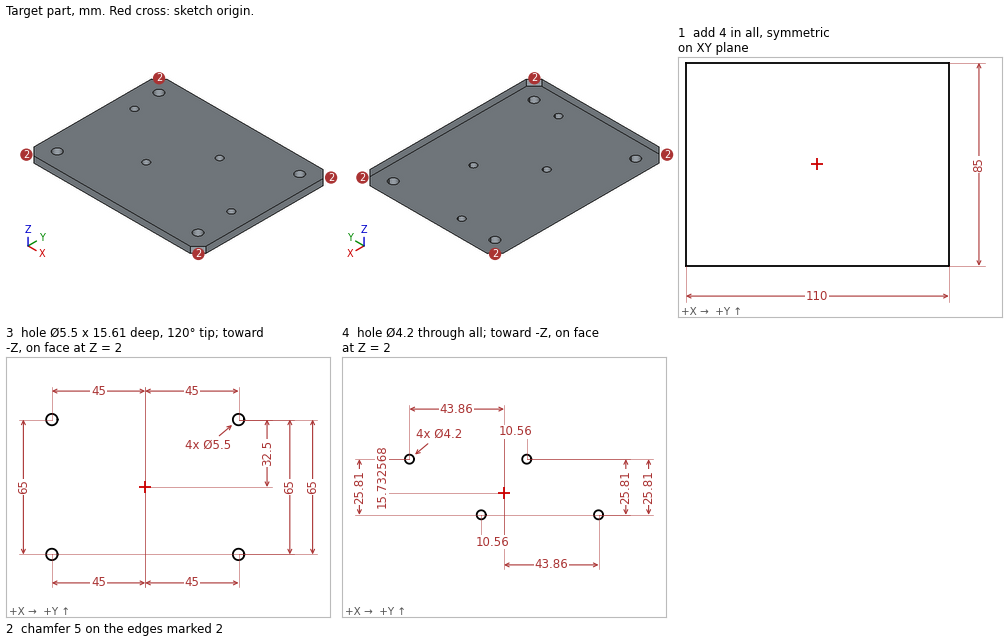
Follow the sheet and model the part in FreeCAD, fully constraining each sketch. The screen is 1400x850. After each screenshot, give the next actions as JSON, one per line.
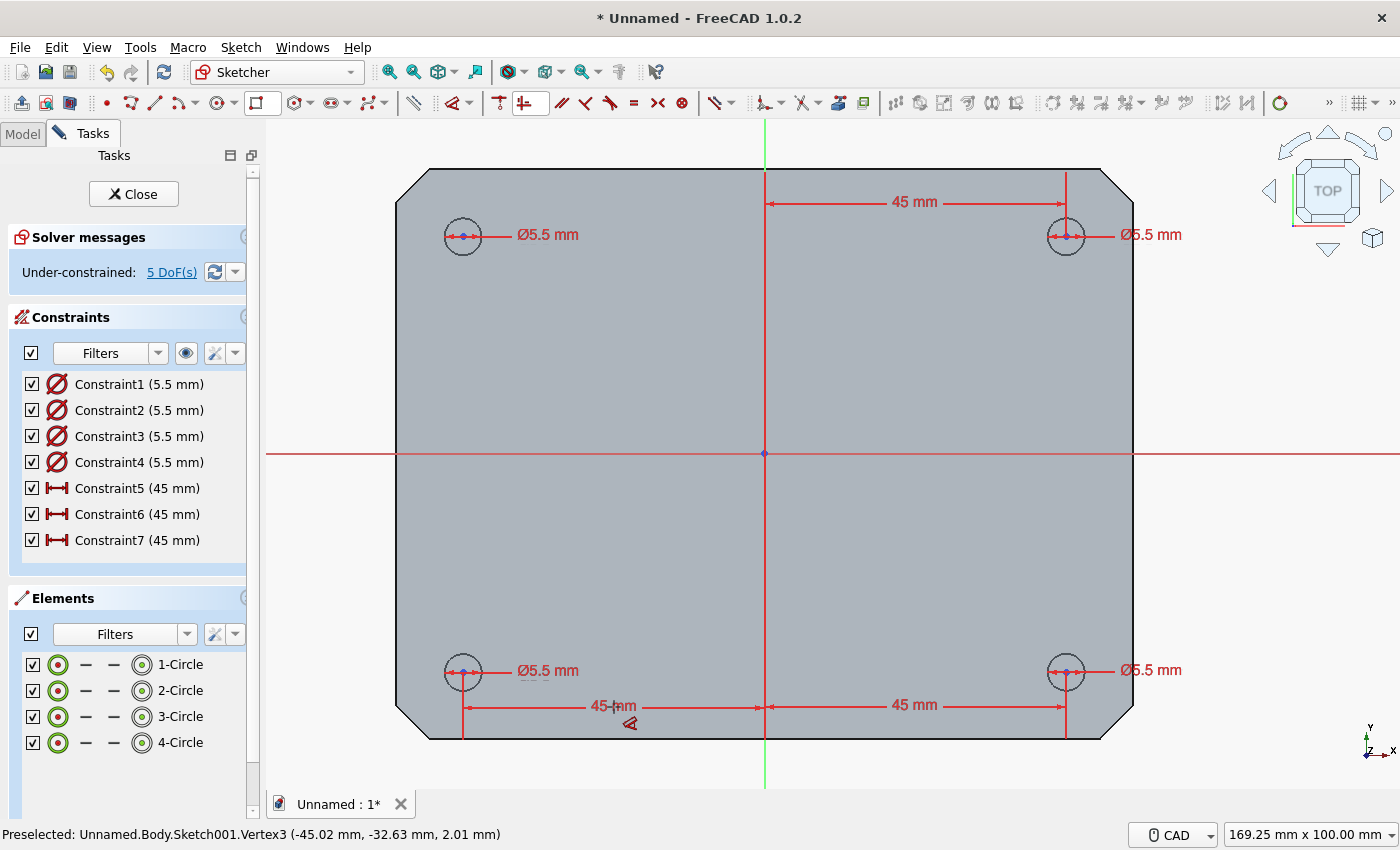
{"action": "left_click", "coordinate": [463, 237]}
{"action": "left_click", "coordinate": [614, 203]}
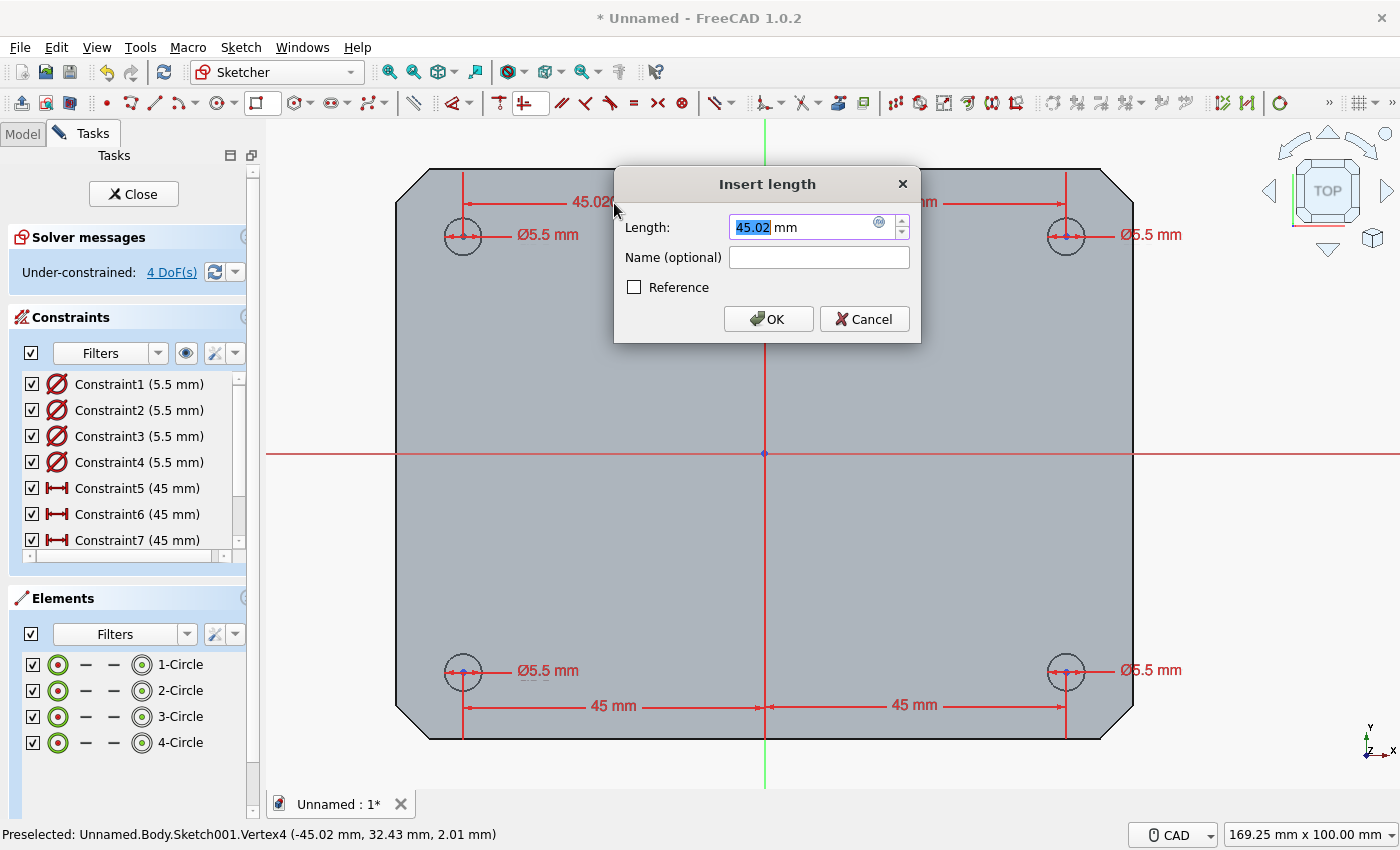
{"action": "type", "text": "45"}
{"action": "key", "text": "Return"}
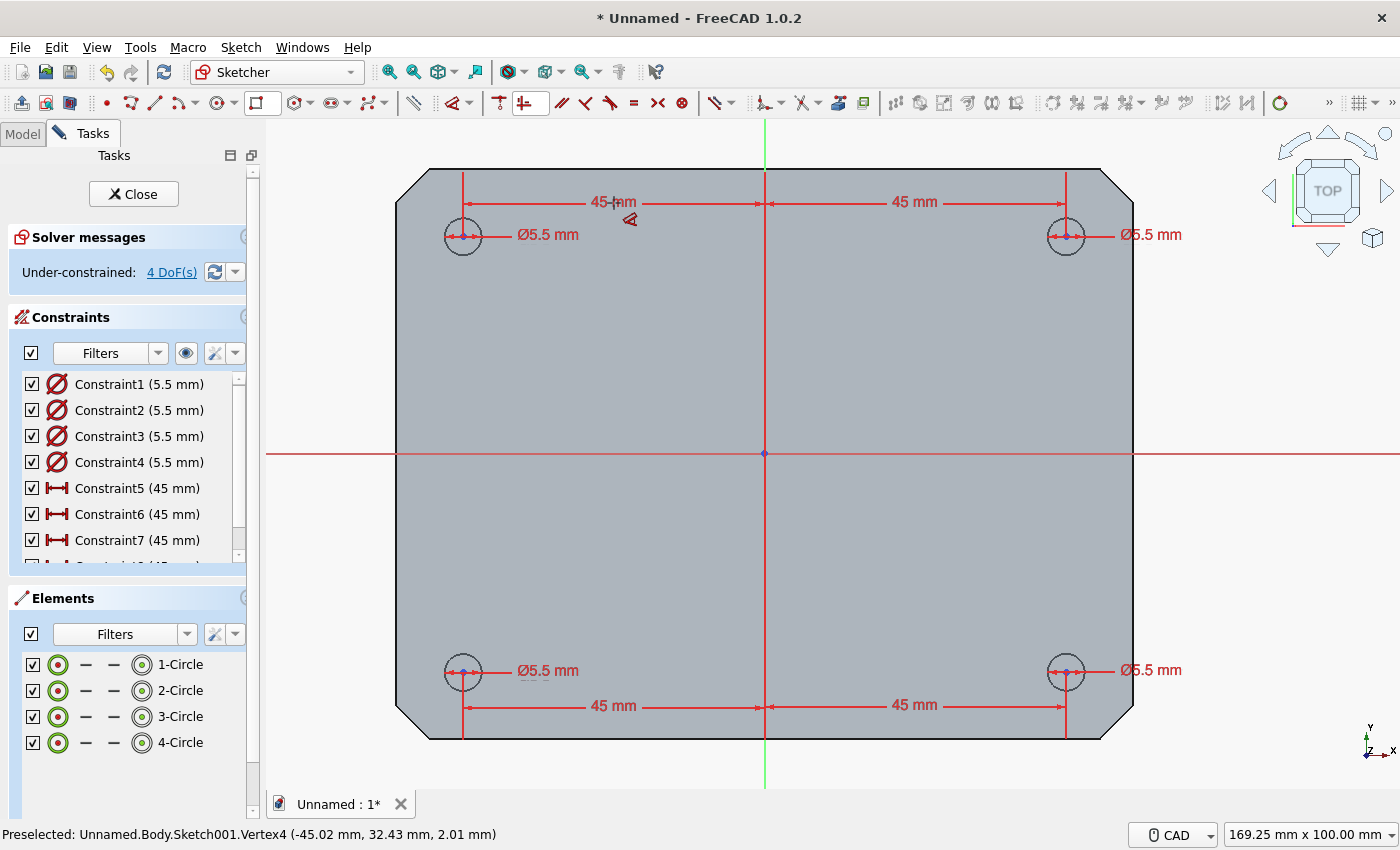
{"action": "left_click", "coordinate": [1066, 237]}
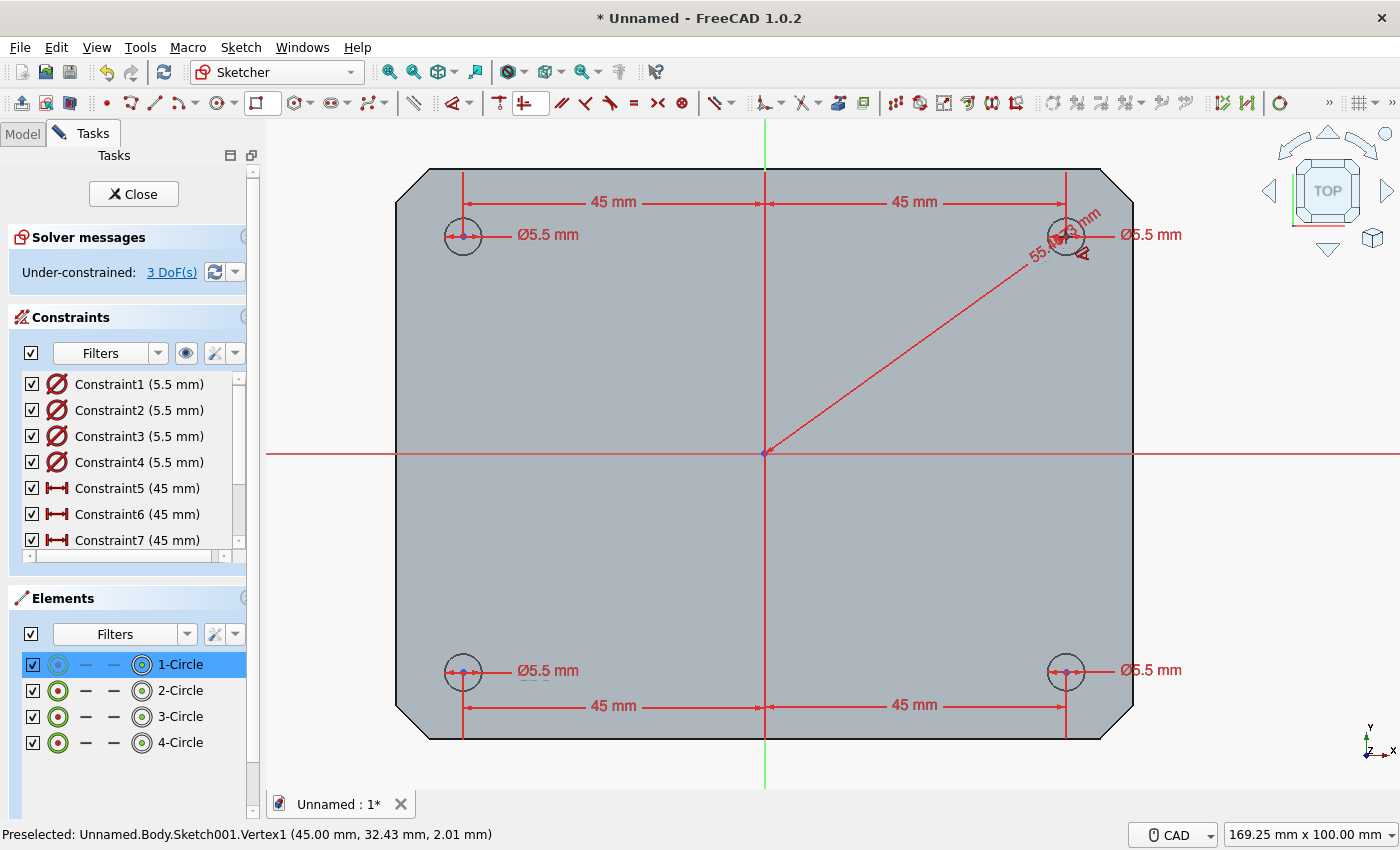
{"action": "left_click", "coordinate": [1066, 672]}
{"action": "left_click", "coordinate": [1100, 354]}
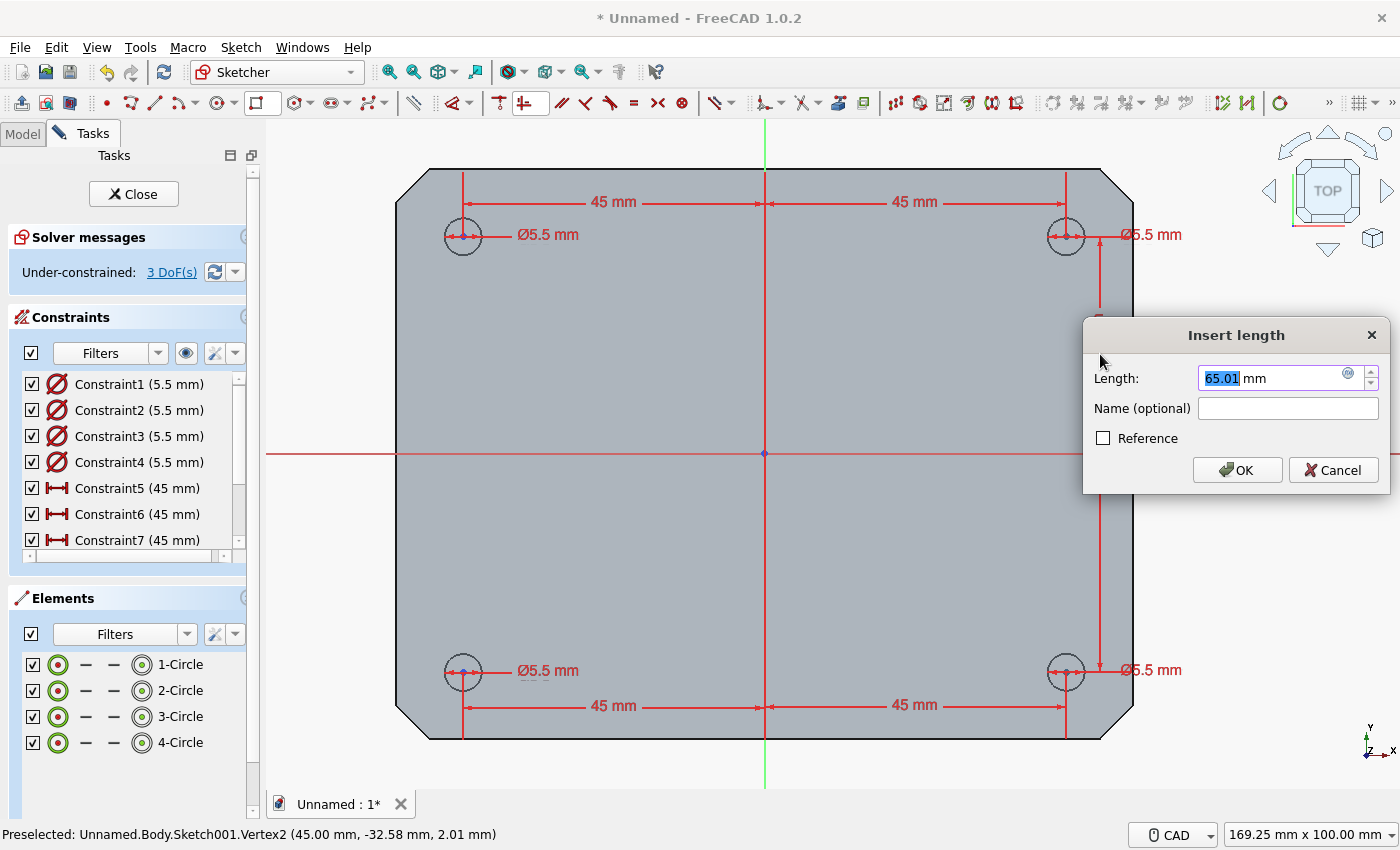
{"action": "type", "text": "65"}
{"action": "key", "text": "Return"}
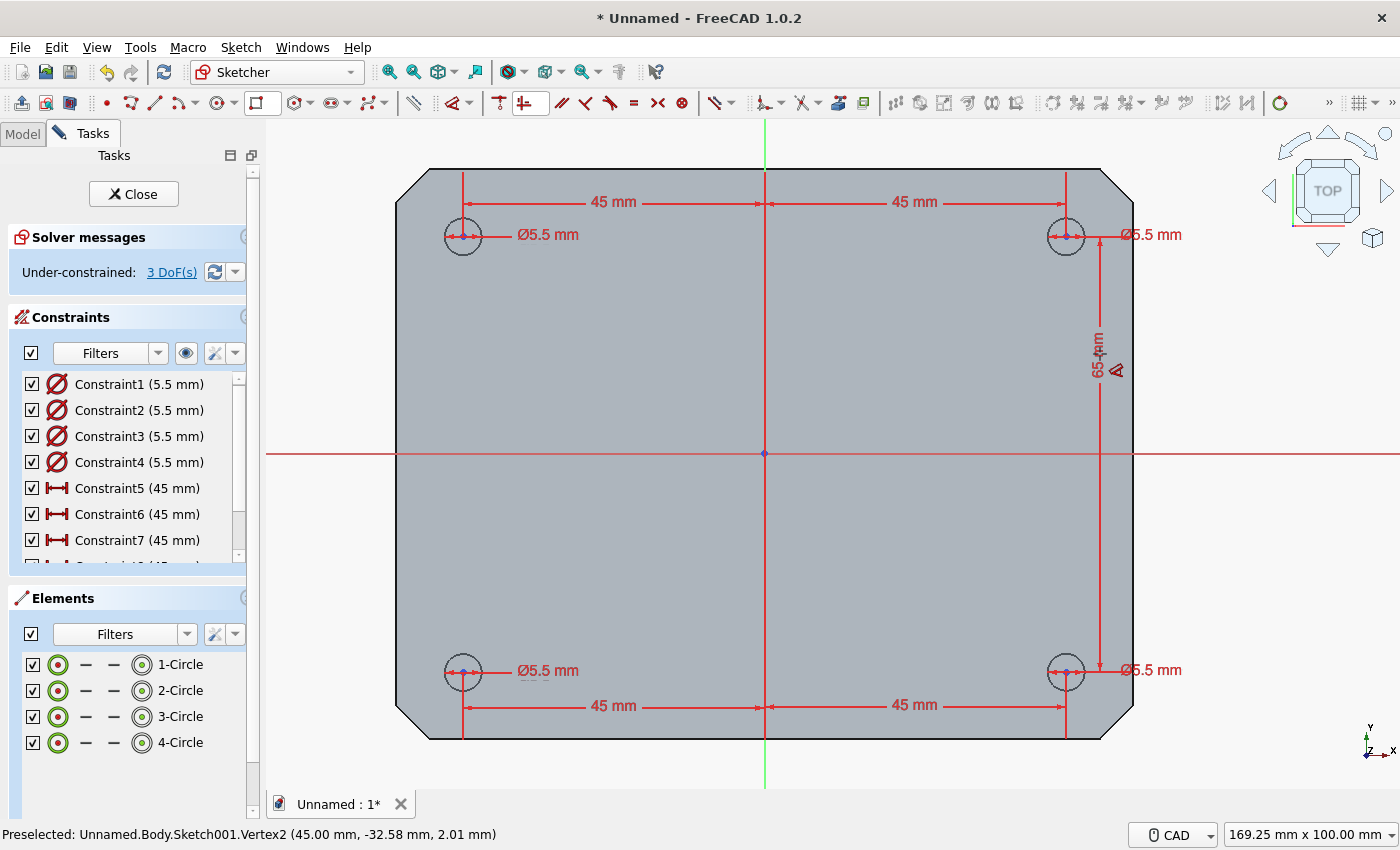
{"action": "left_click", "coordinate": [1066, 237]}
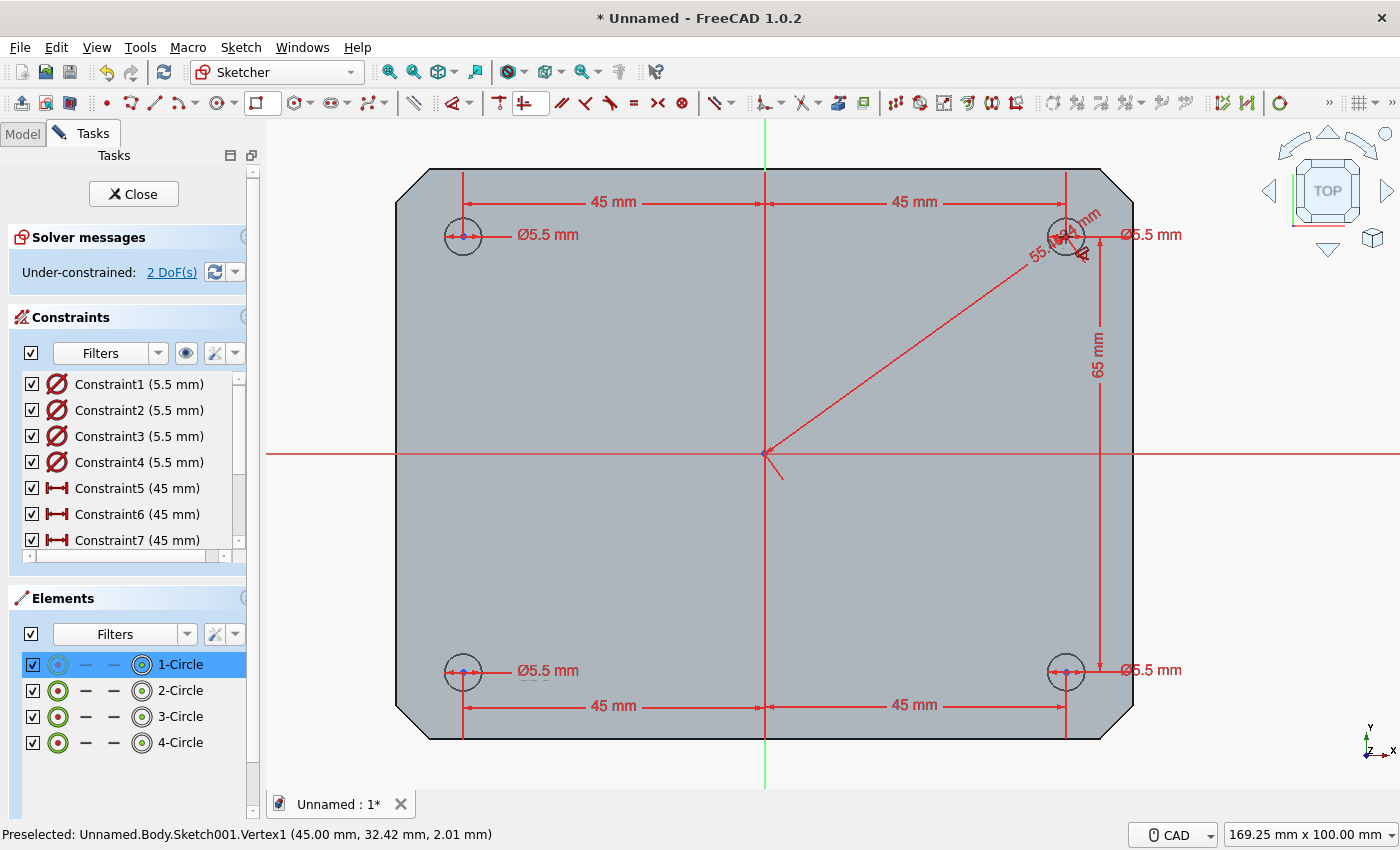
{"action": "left_click", "coordinate": [463, 673]}
{"action": "left_click", "coordinate": [429, 354]}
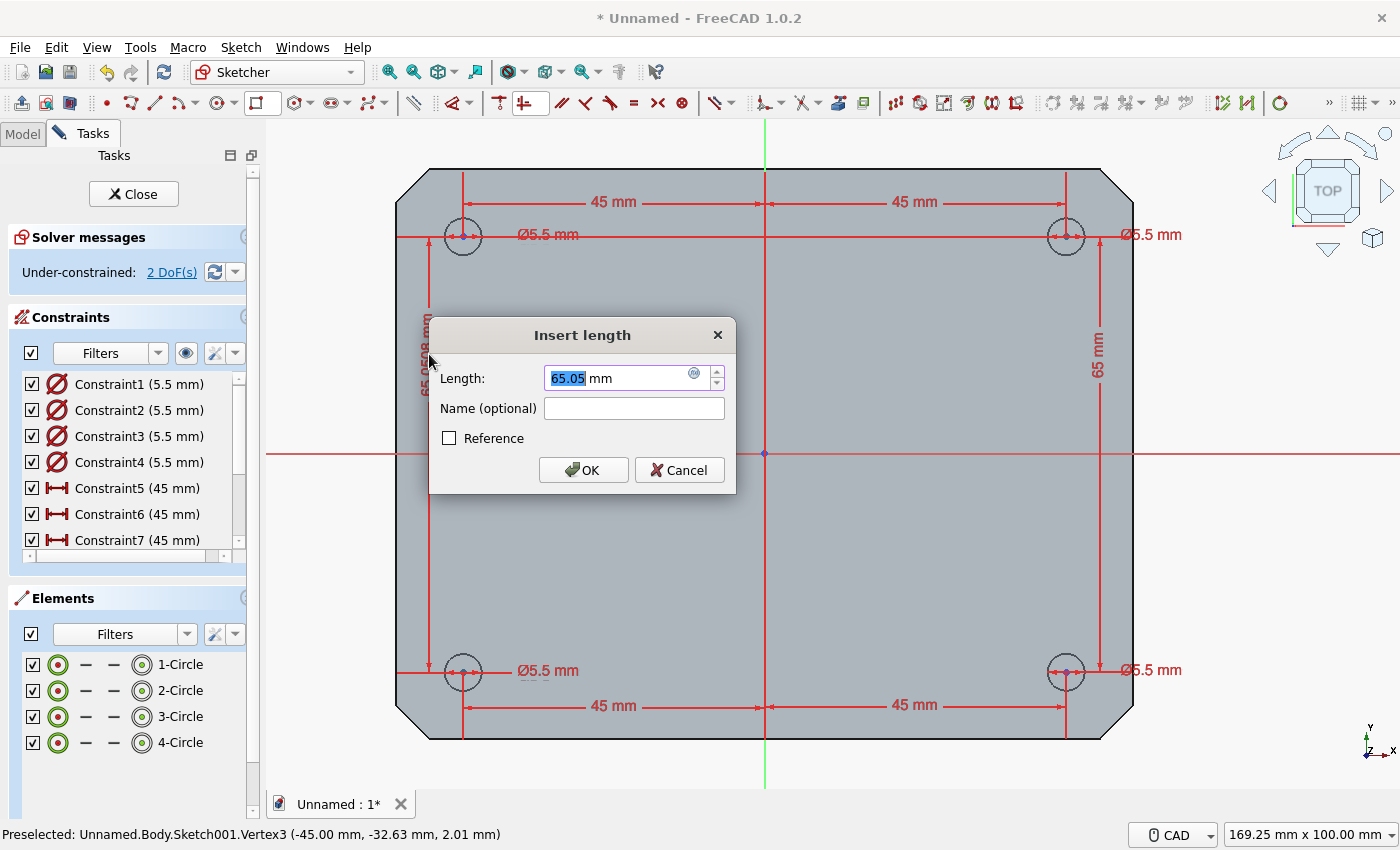
{"action": "type", "text": "65"}
{"action": "key", "text": "Return"}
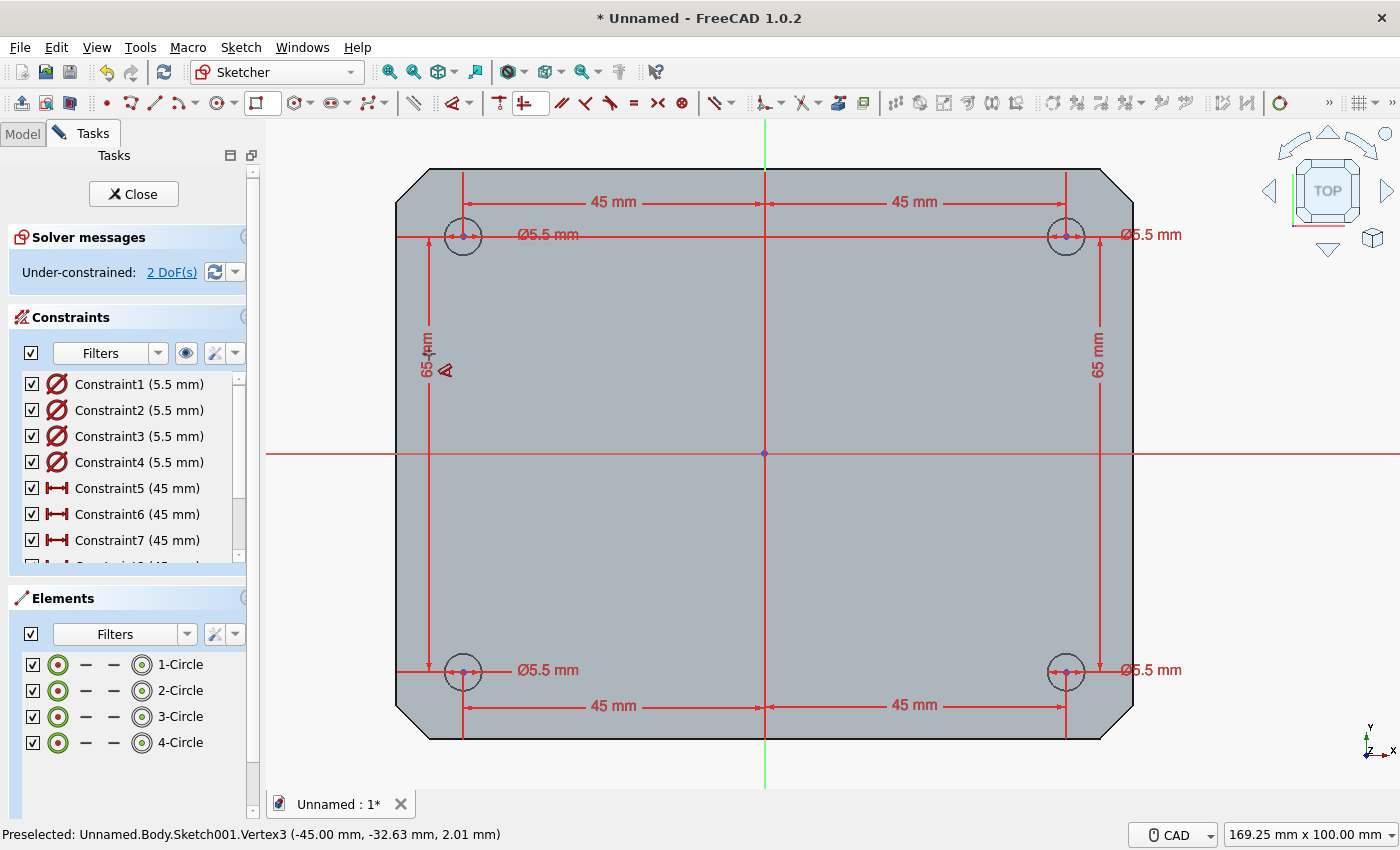
{"action": "left_click", "coordinate": [463, 672]}